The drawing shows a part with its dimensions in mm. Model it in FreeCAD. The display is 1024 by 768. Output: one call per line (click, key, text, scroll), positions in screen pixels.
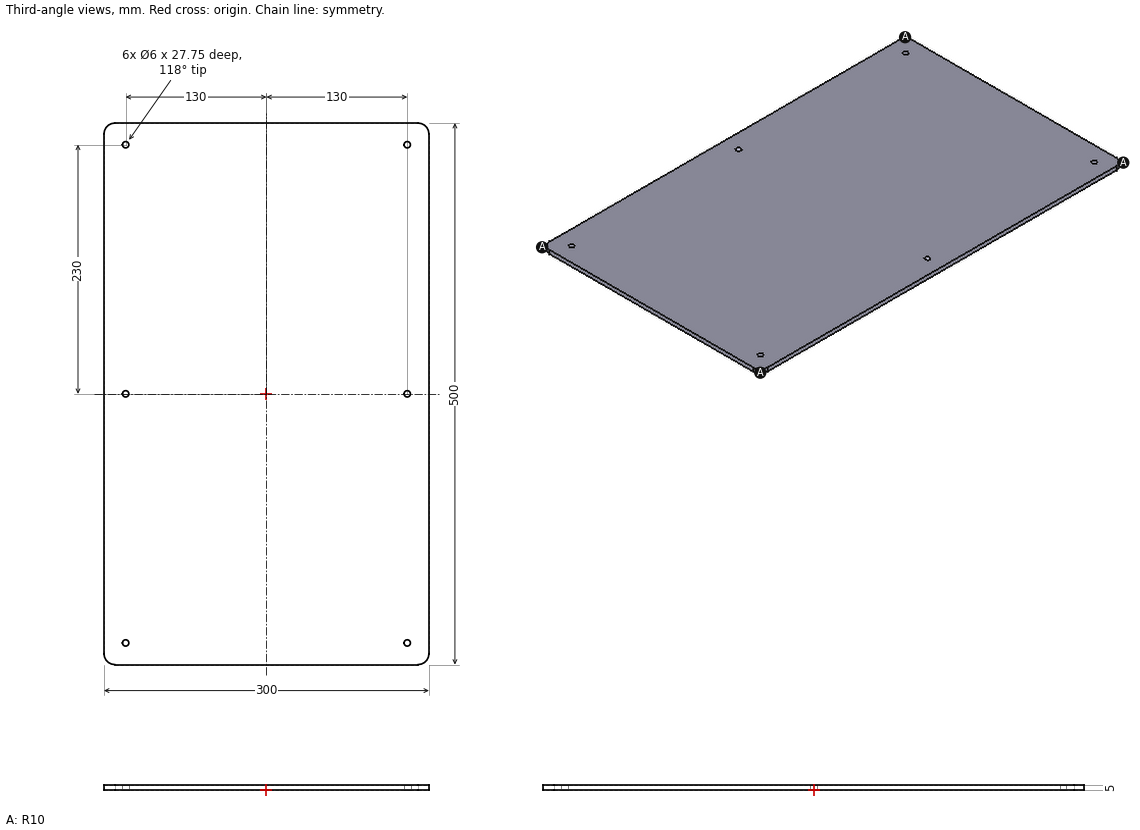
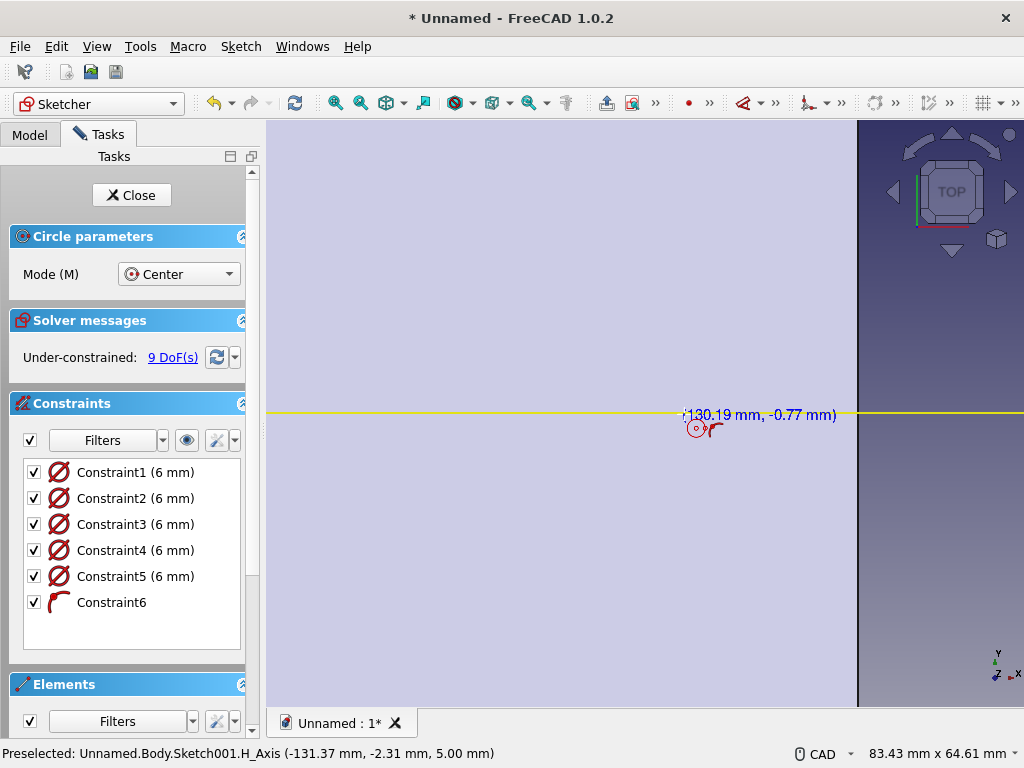
scroll(684, 414, down, 12)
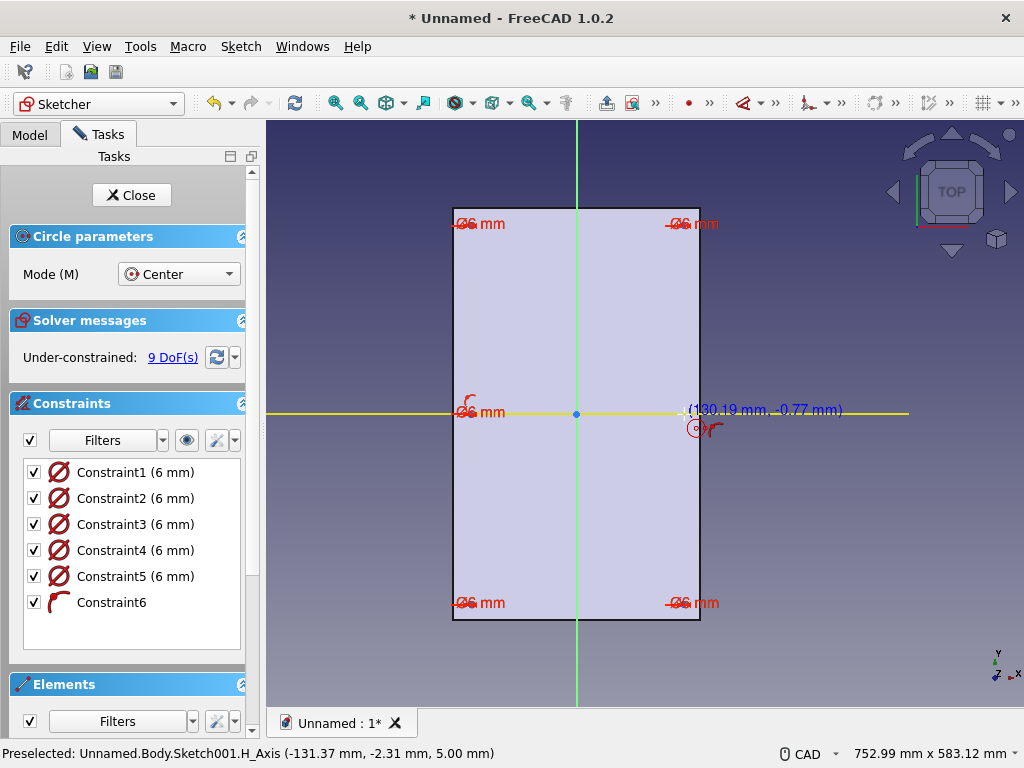
click(684, 414)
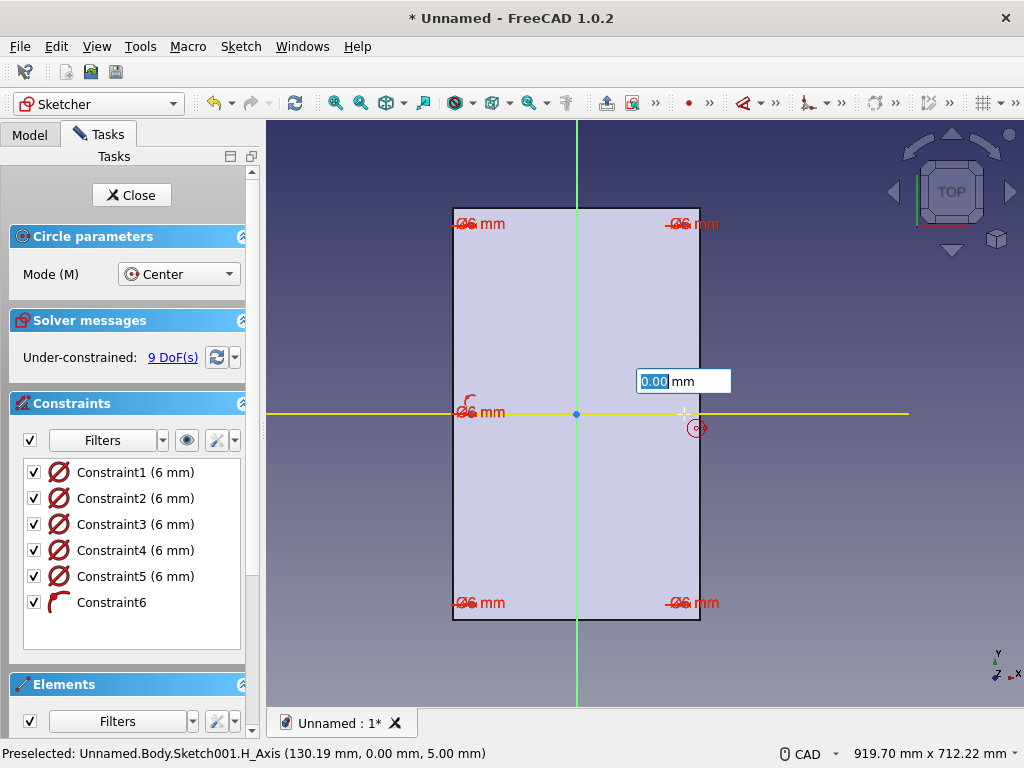
scroll(685, 412, up, 10)
move(679, 409)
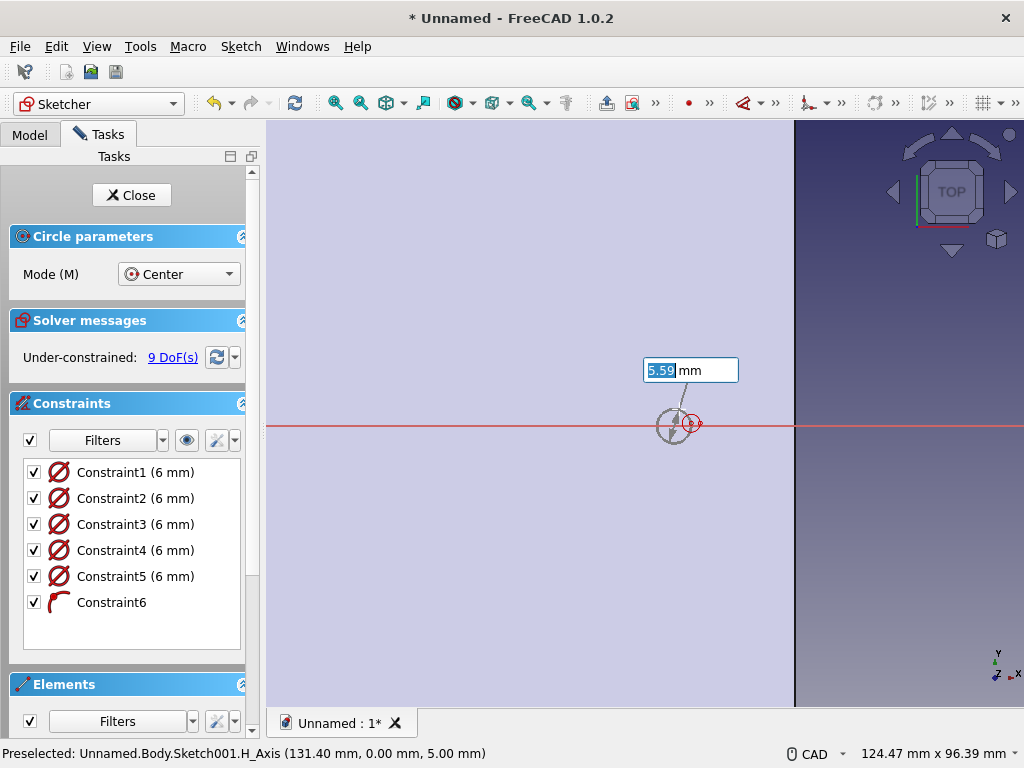
text(6)
key(Return)
key(Escape)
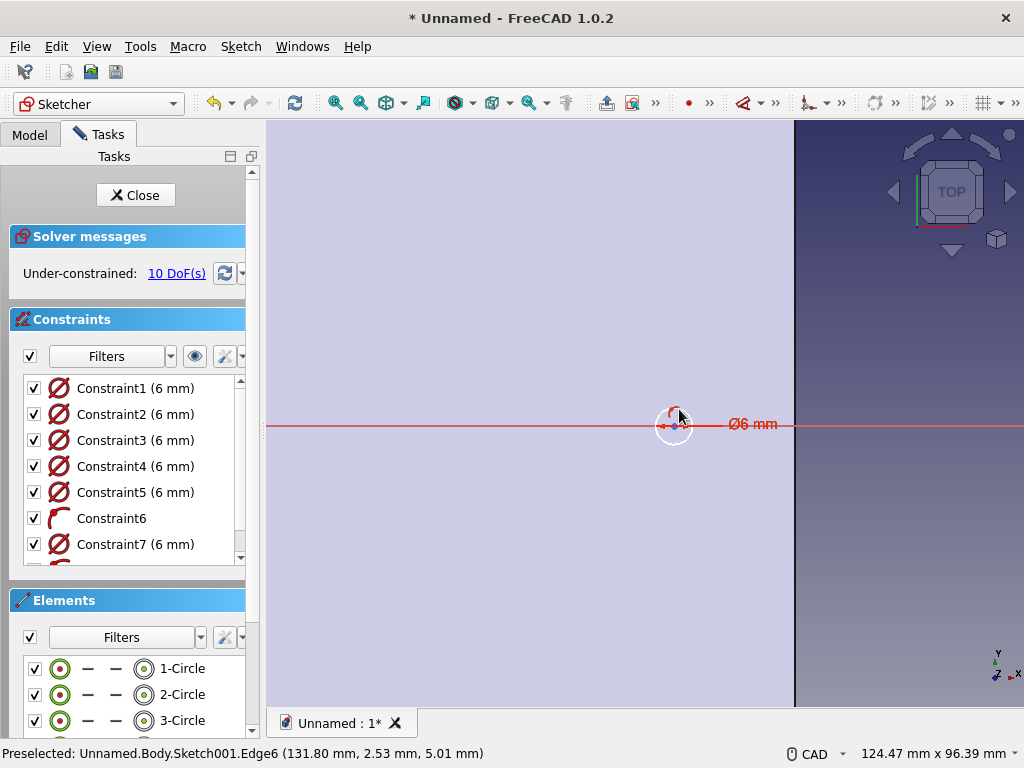
scroll(685, 411, down, 10)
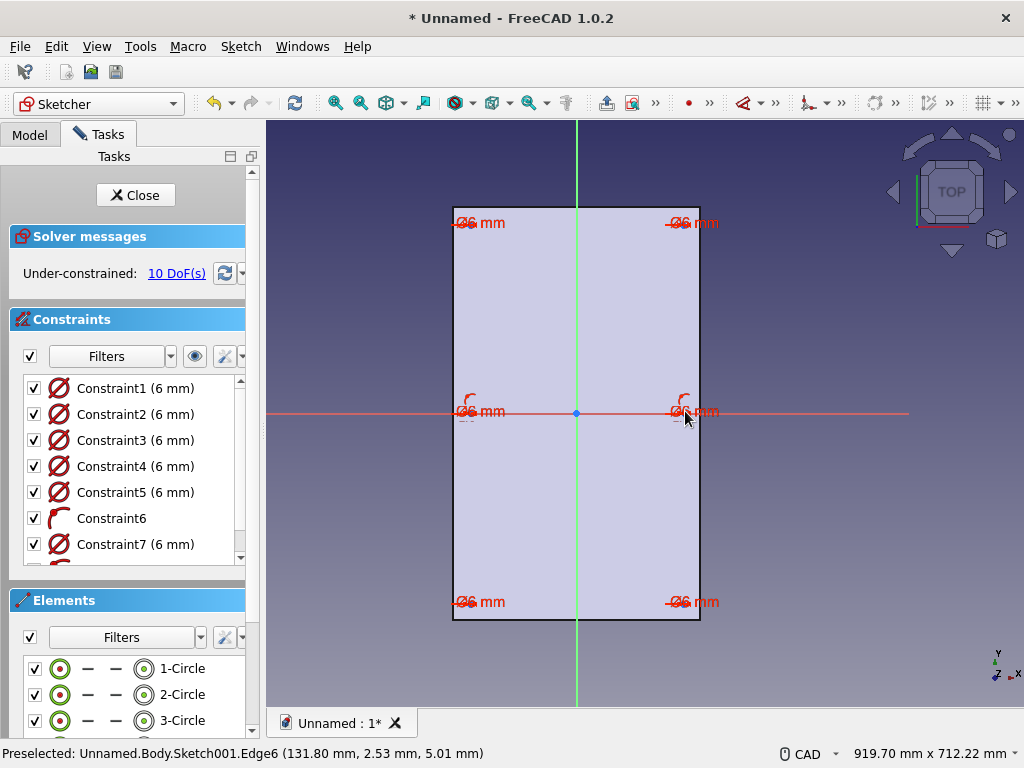
click(470, 225)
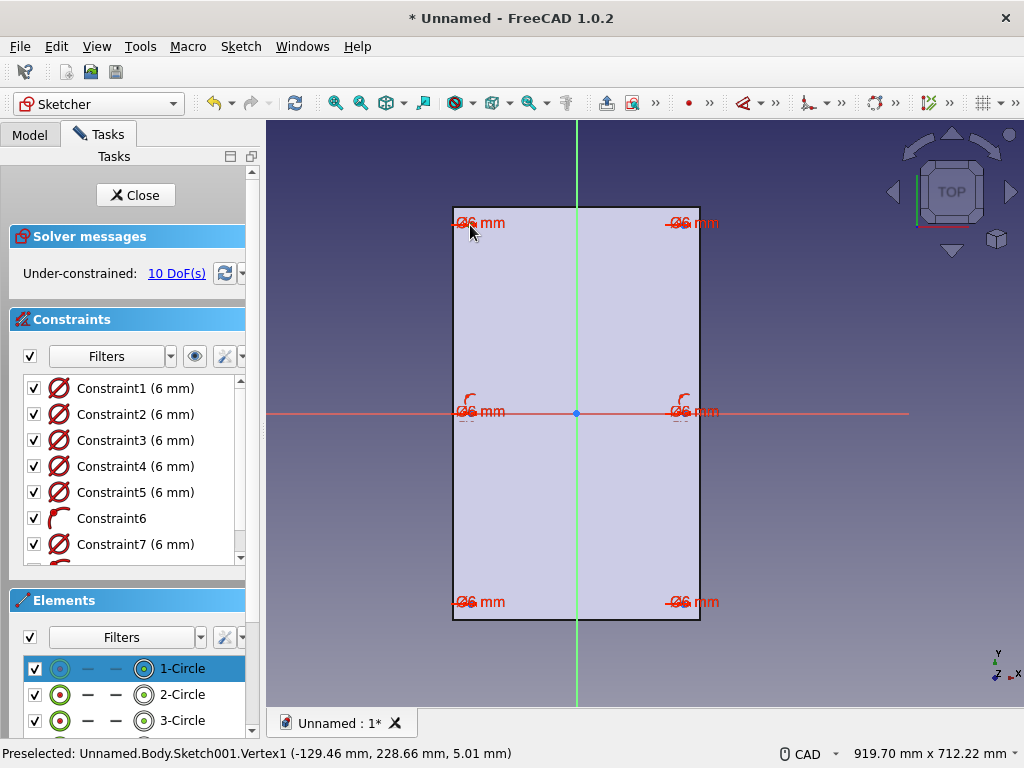
click(684, 225)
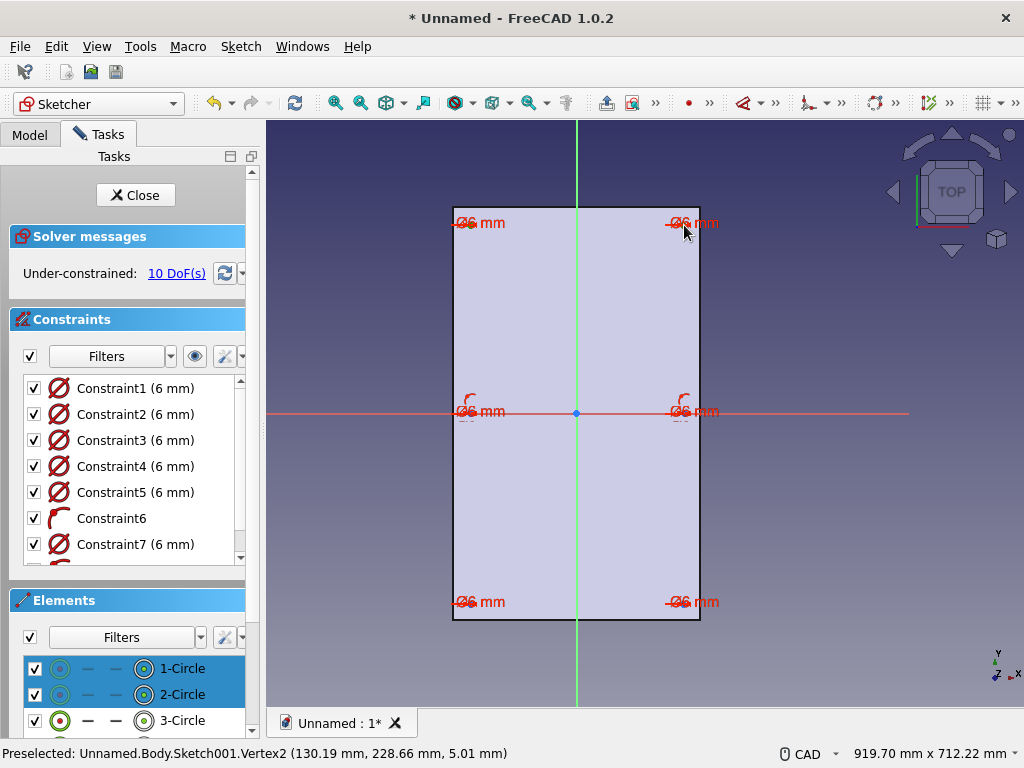
click(577, 641)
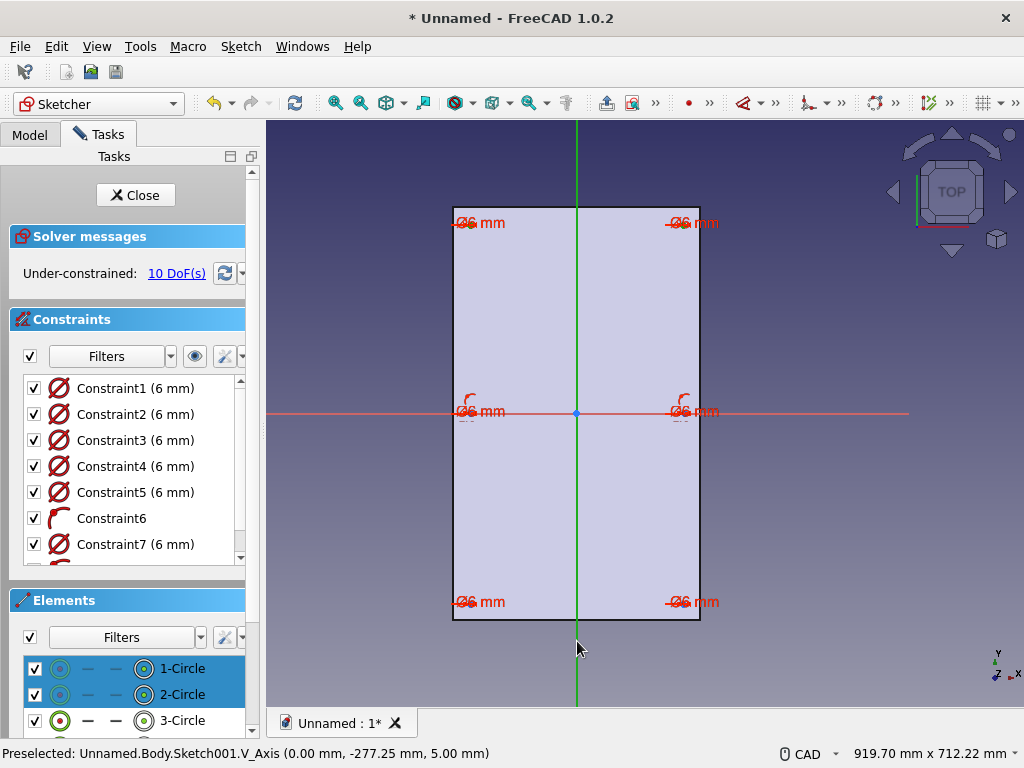
key(s)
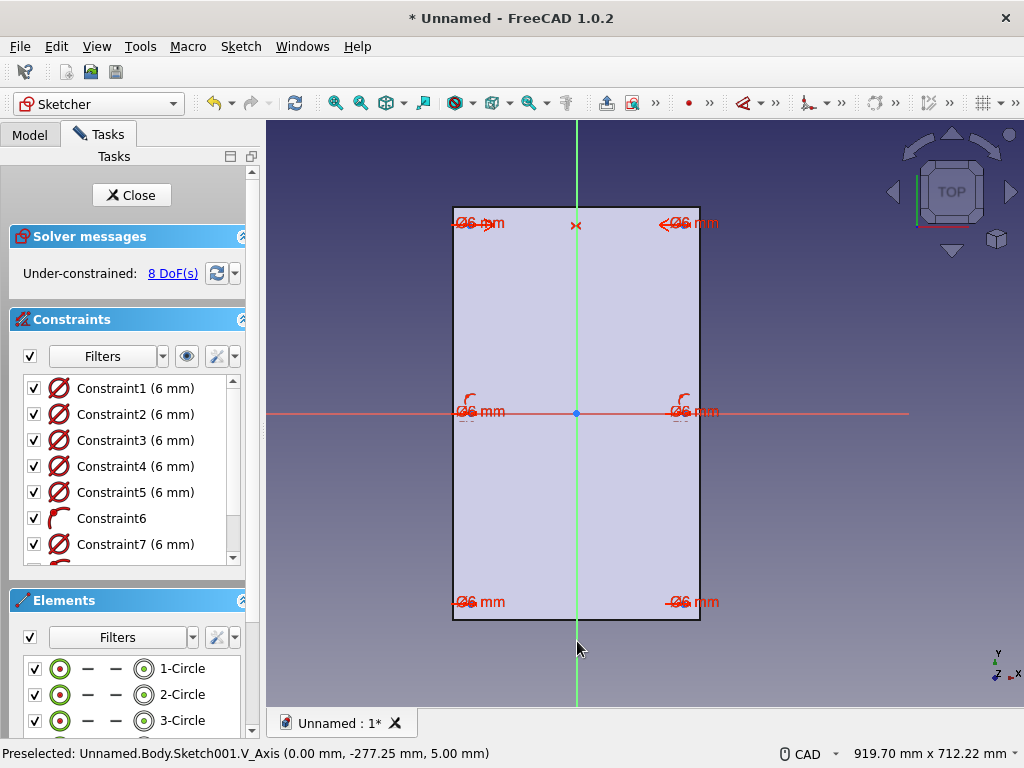
click(684, 225)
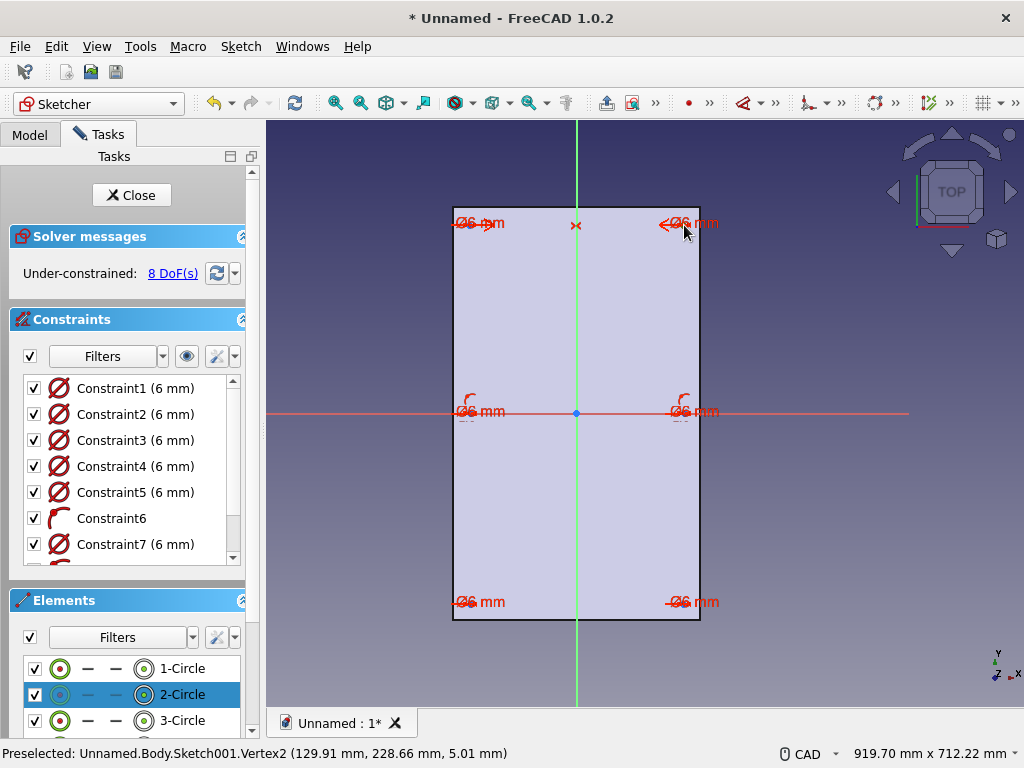
click(684, 604)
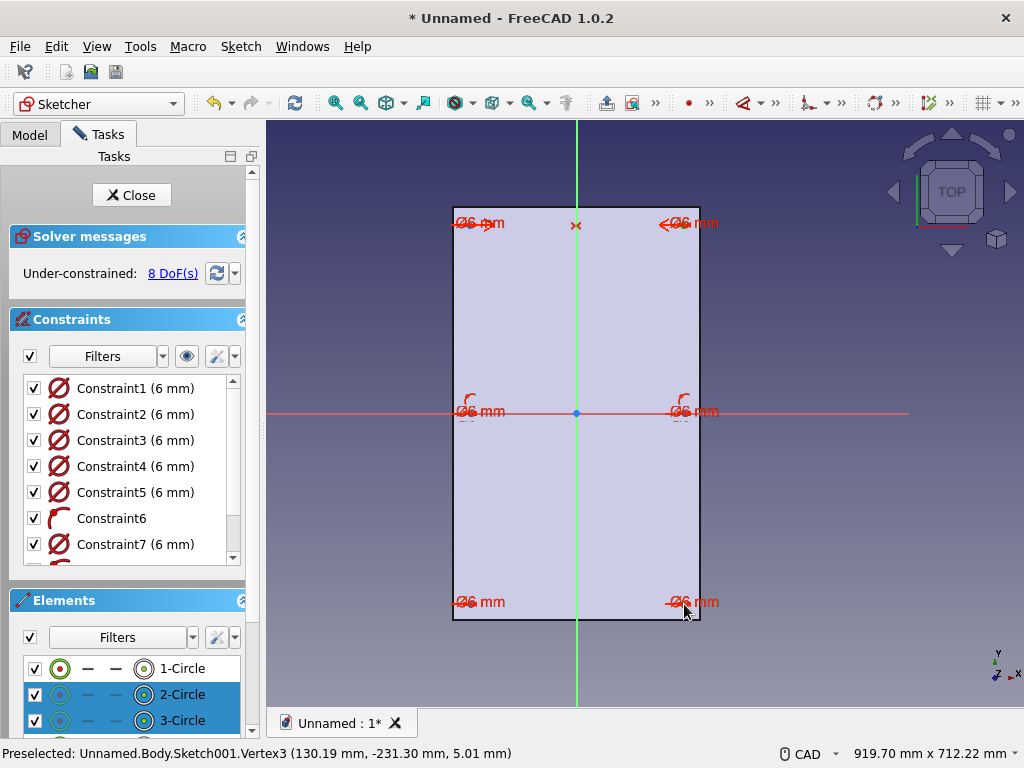
click(334, 413)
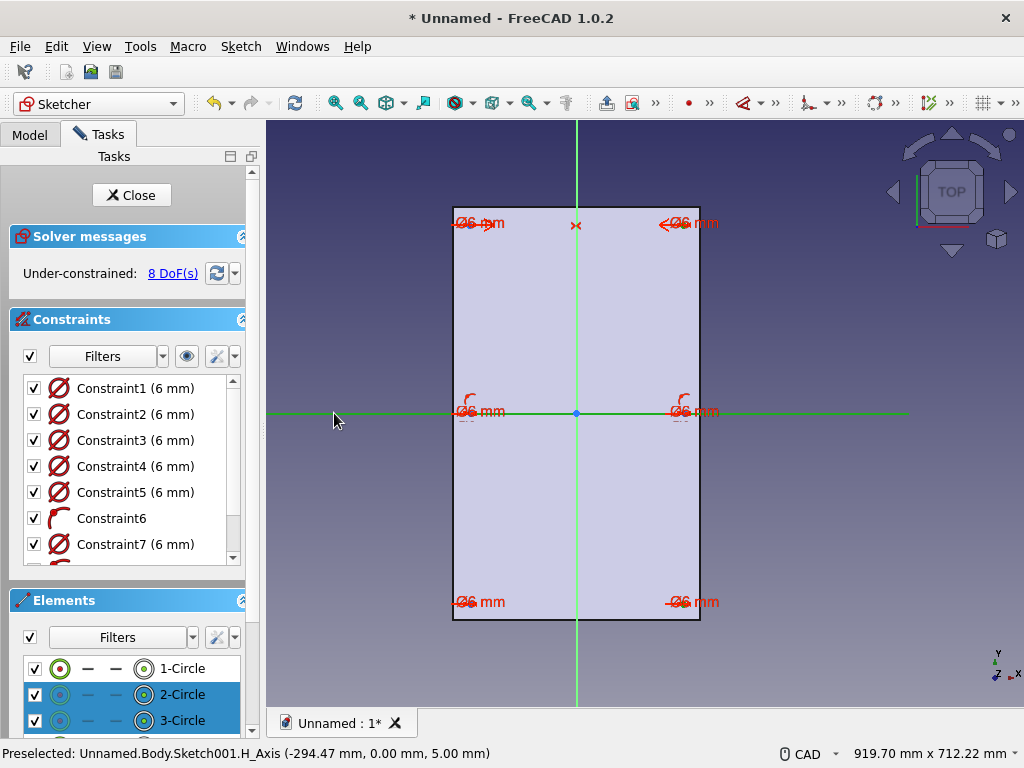
key(s)